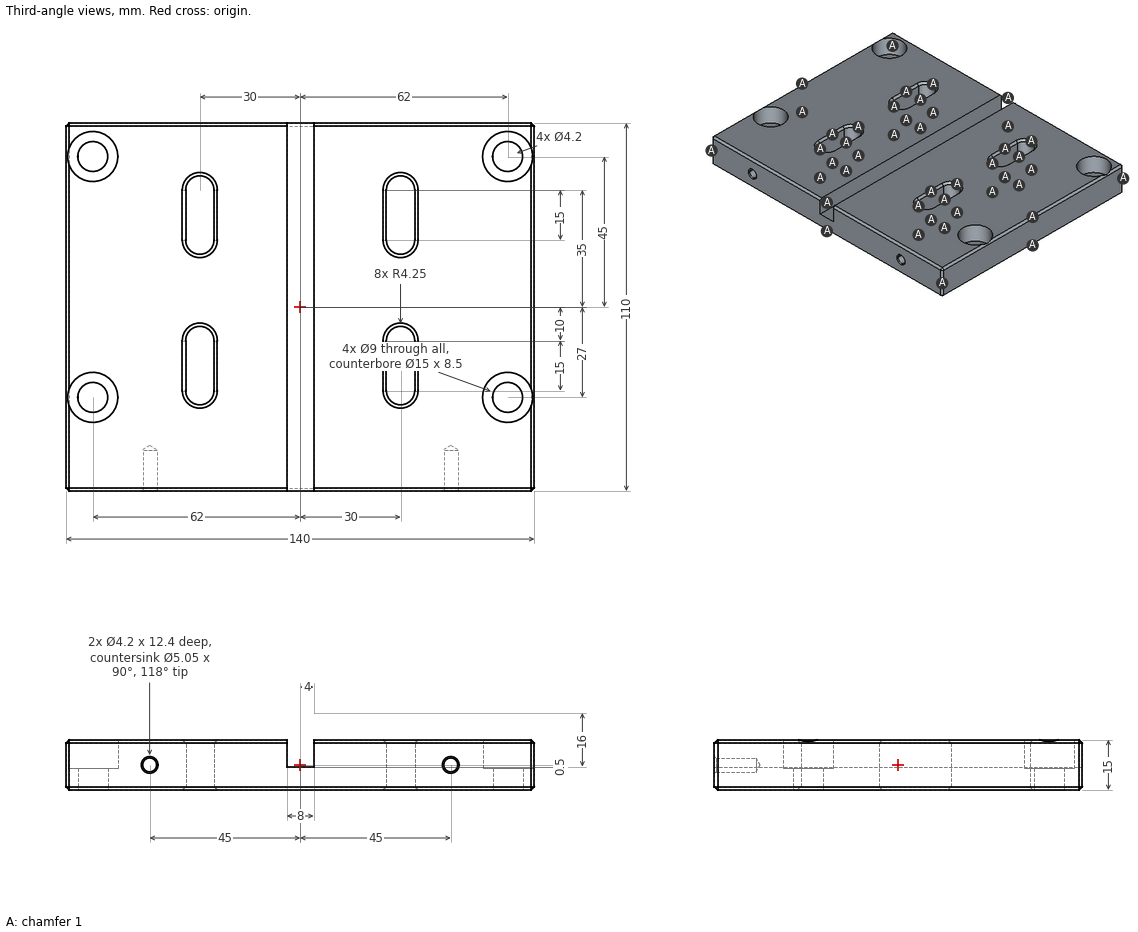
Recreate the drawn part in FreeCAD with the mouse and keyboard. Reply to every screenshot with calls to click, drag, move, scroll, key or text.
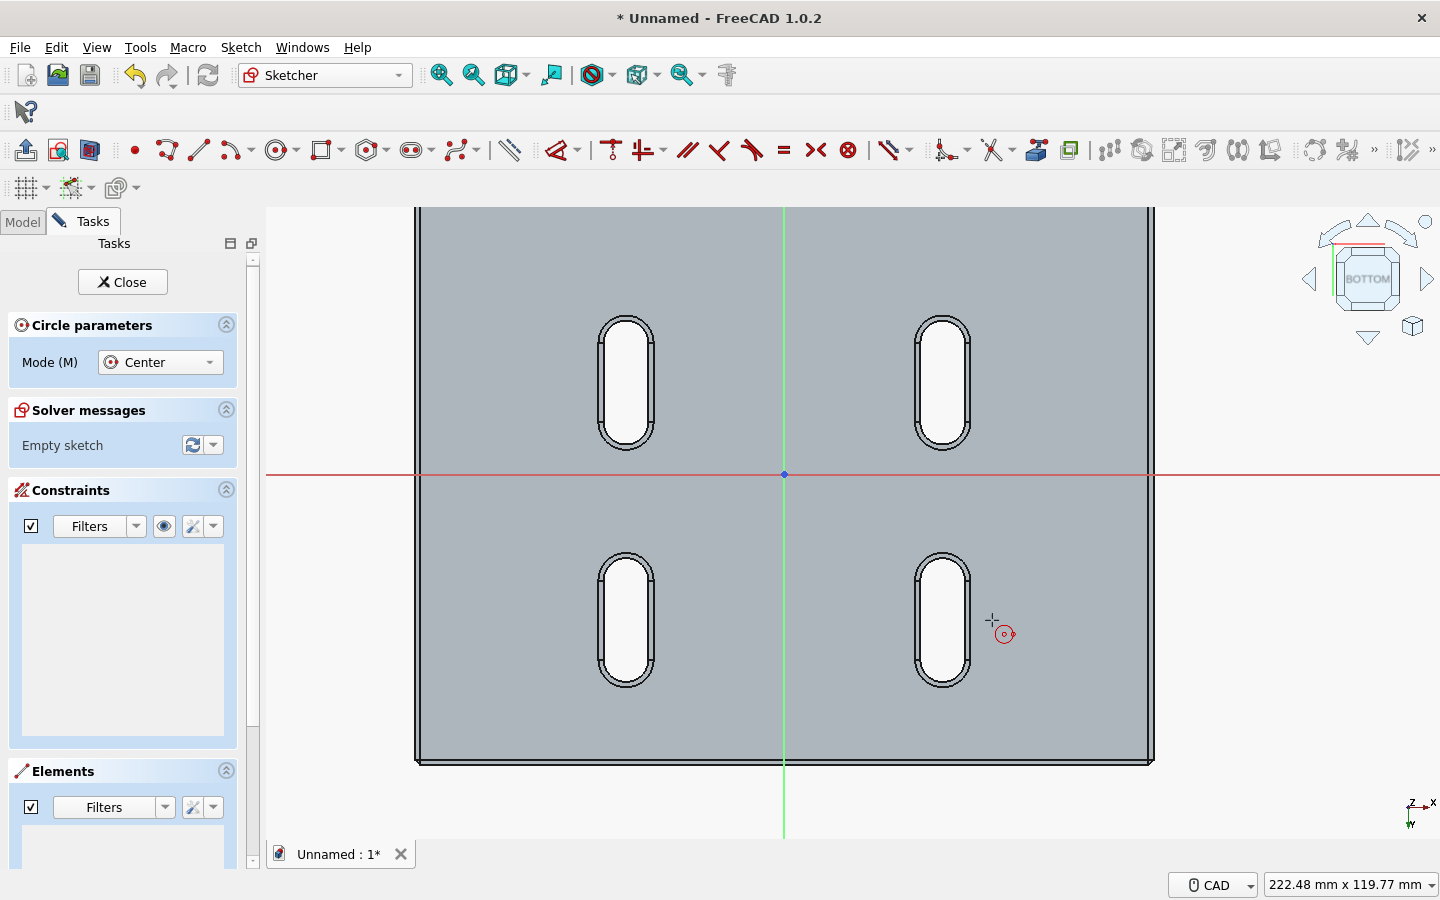
scroll(1111, 712, up, 4)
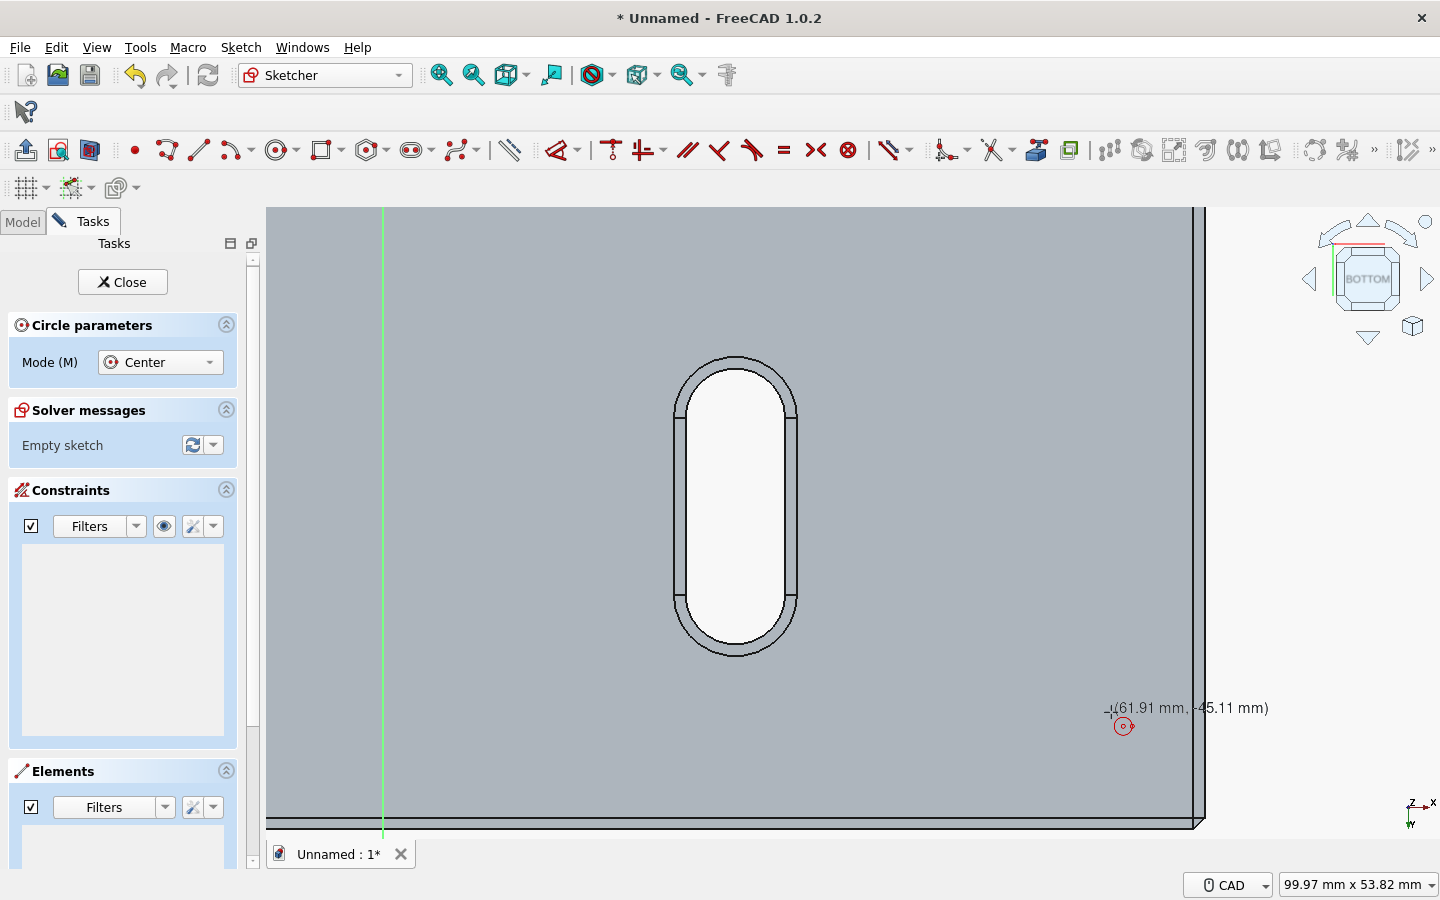
click(1111, 712)
click(1129, 695)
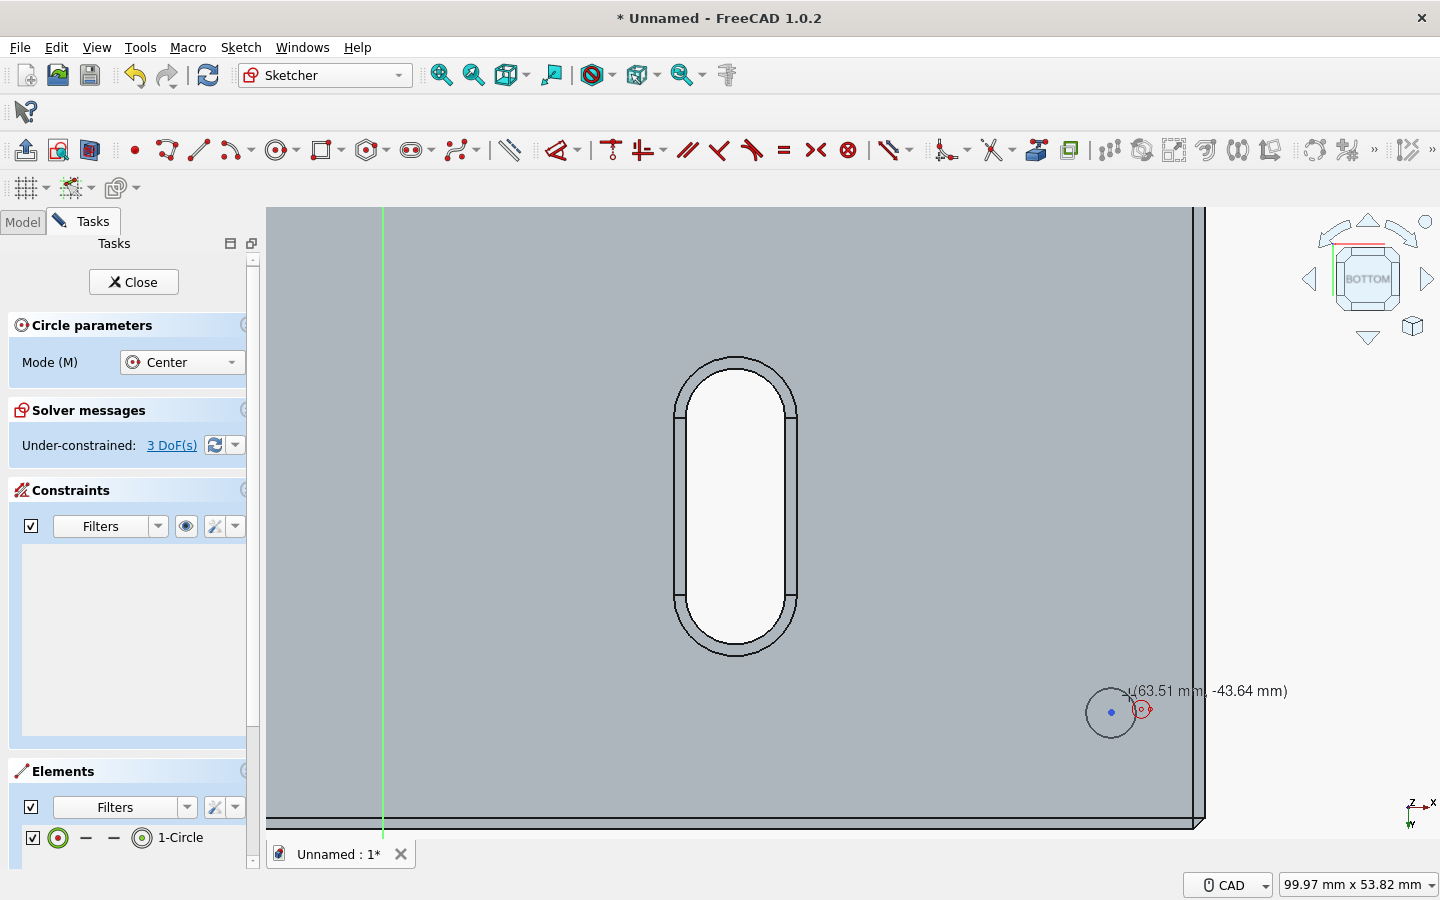
scroll(1112, 714, down, 4)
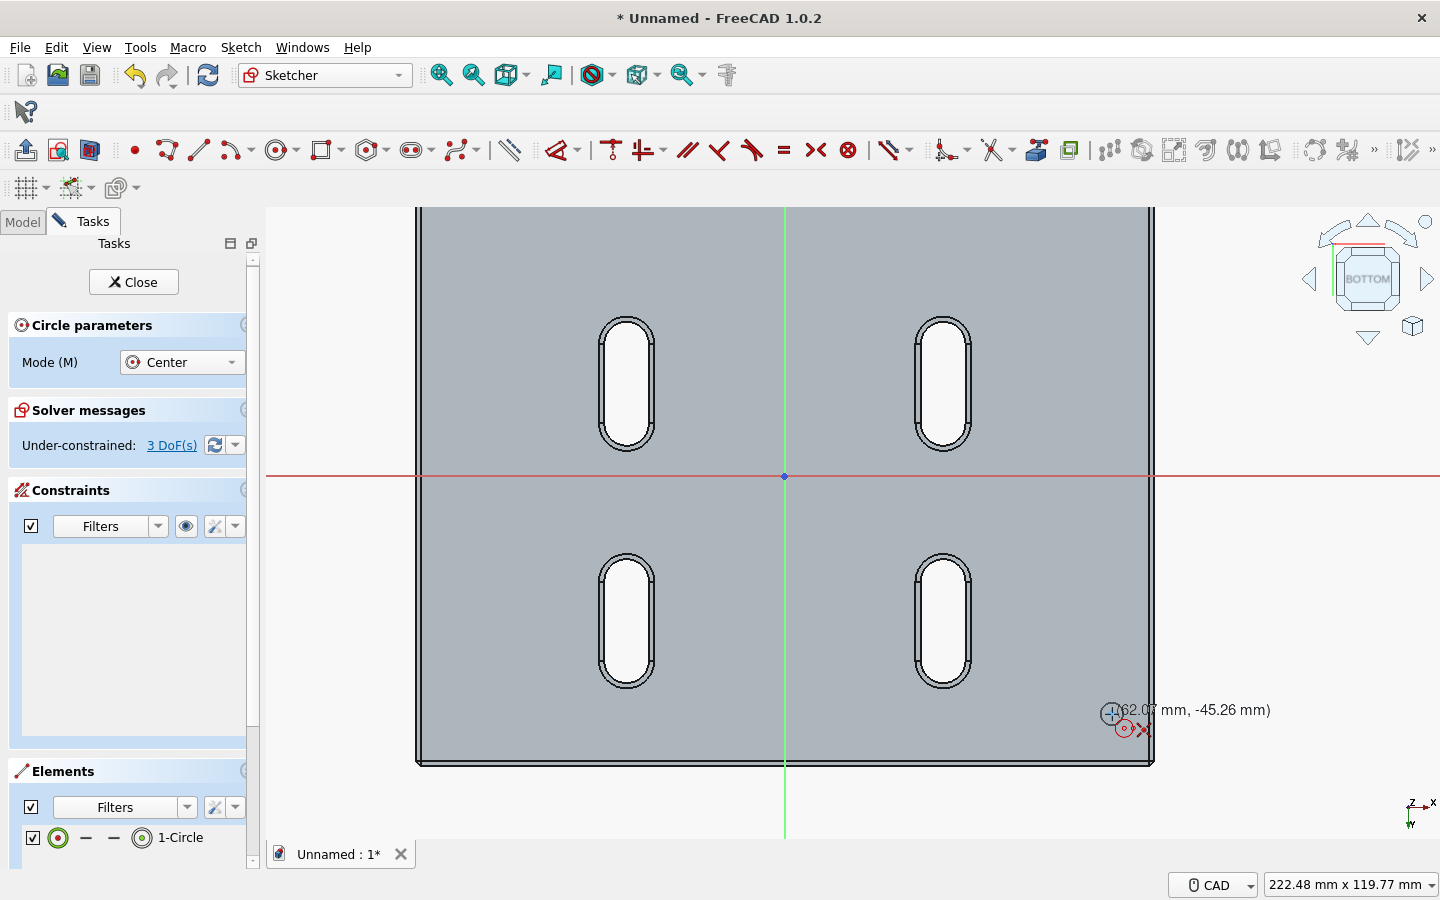
scroll(1112, 334, up, 4)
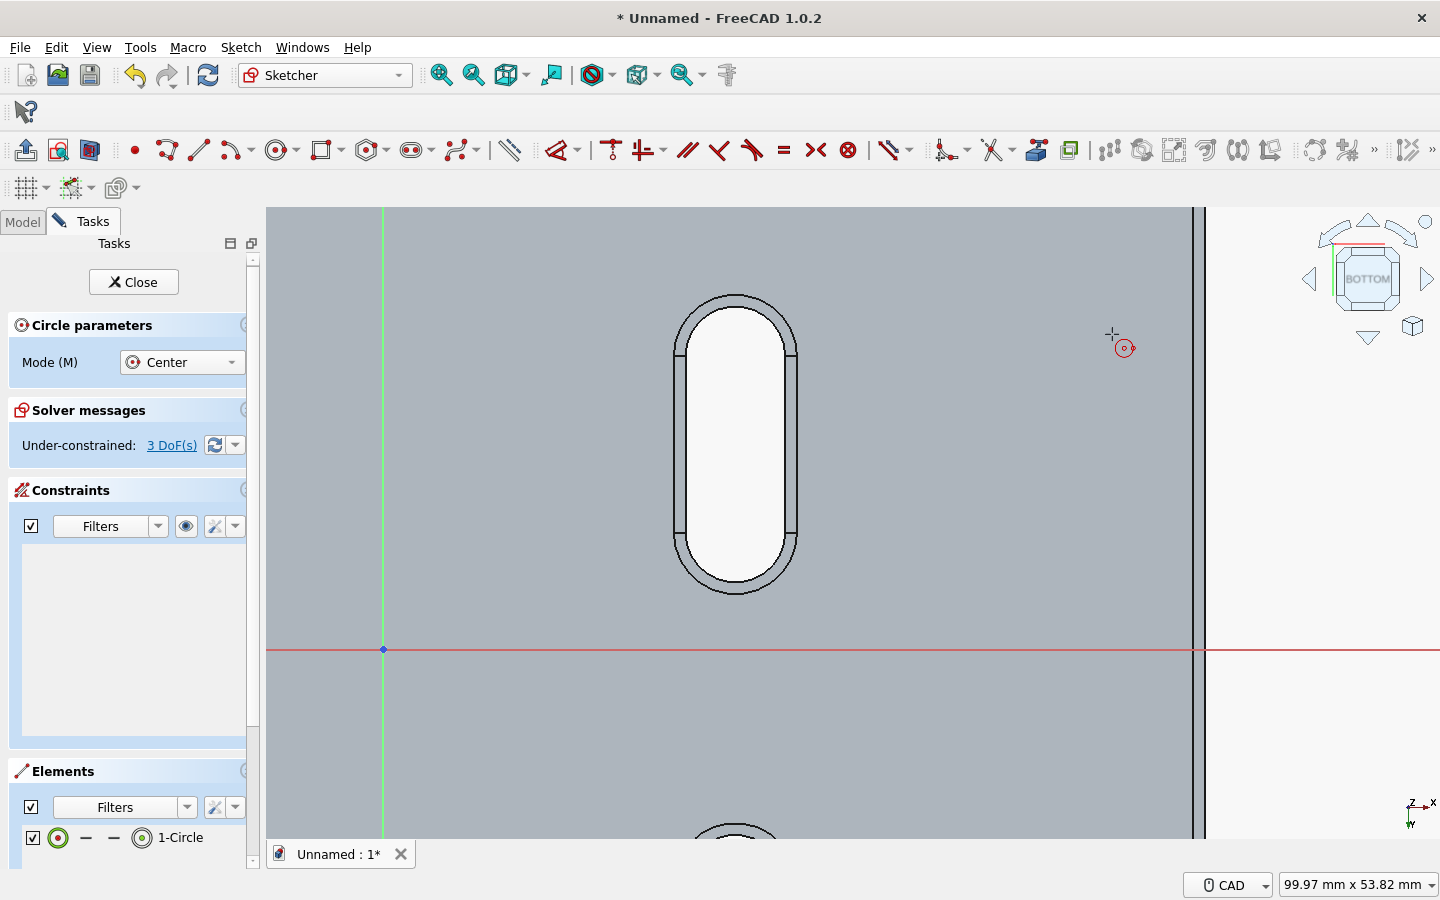
click(1111, 333)
click(1129, 315)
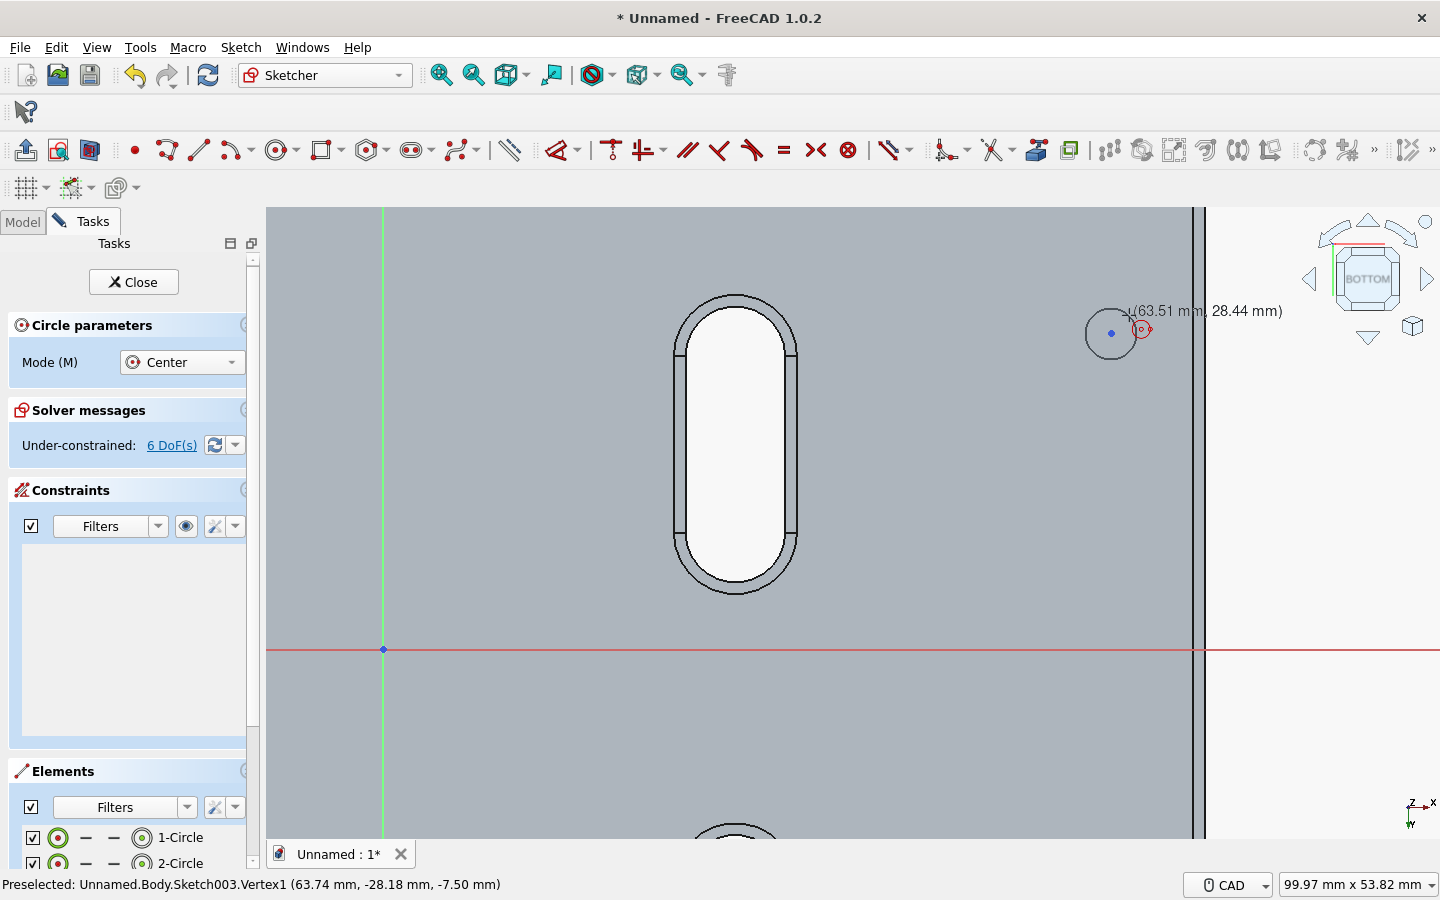
scroll(1112, 333, down, 4)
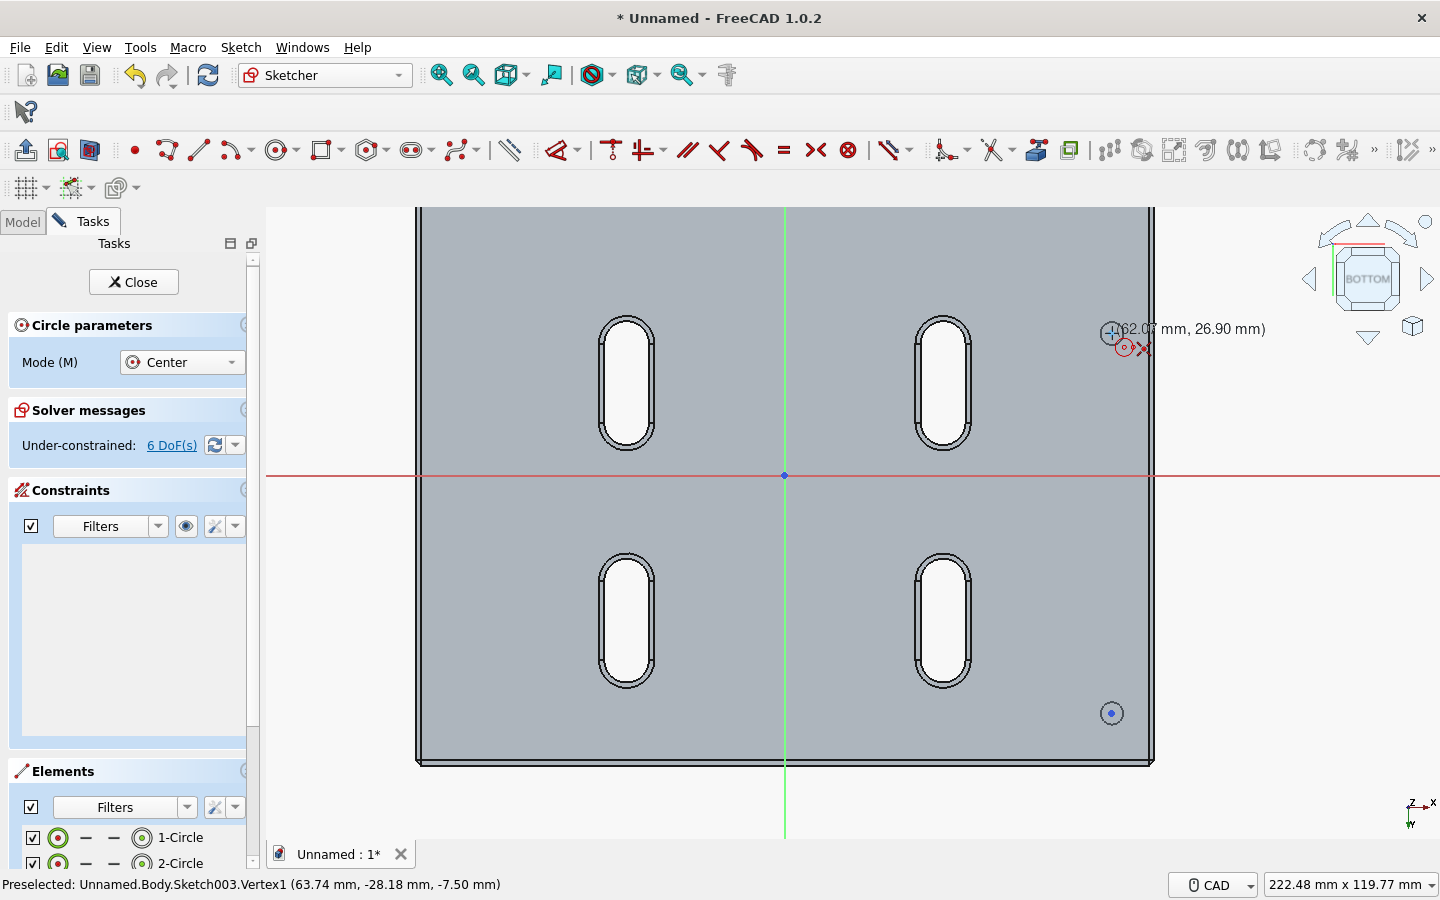
scroll(458, 333, up, 4)